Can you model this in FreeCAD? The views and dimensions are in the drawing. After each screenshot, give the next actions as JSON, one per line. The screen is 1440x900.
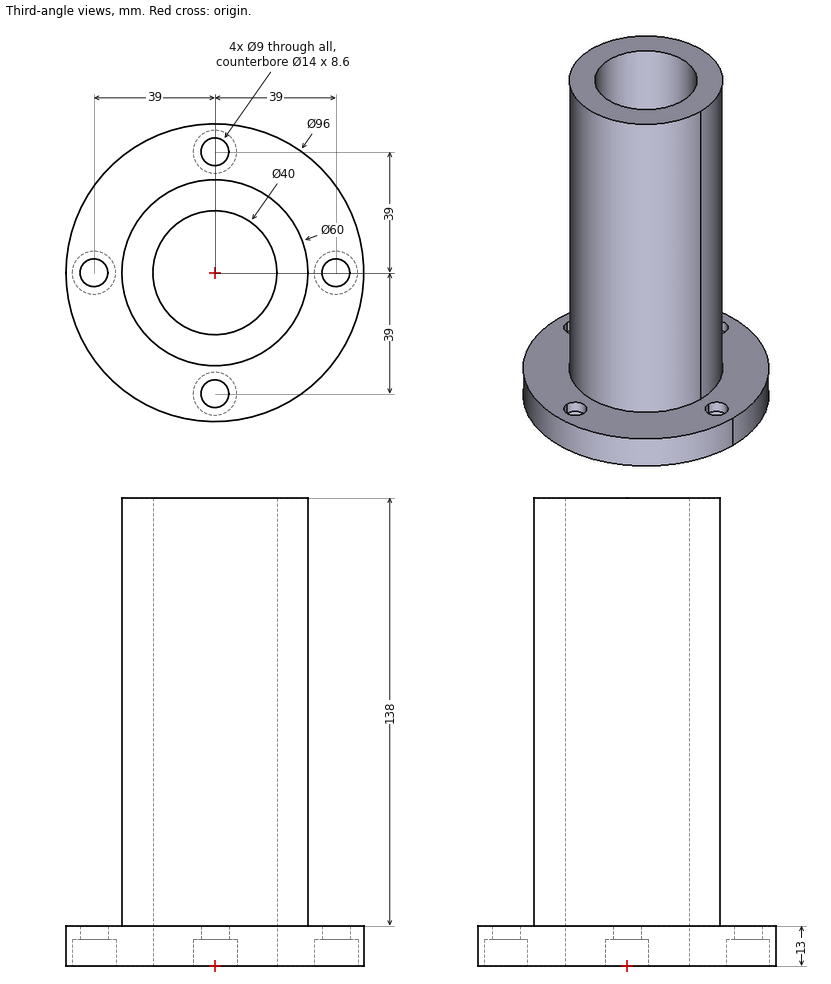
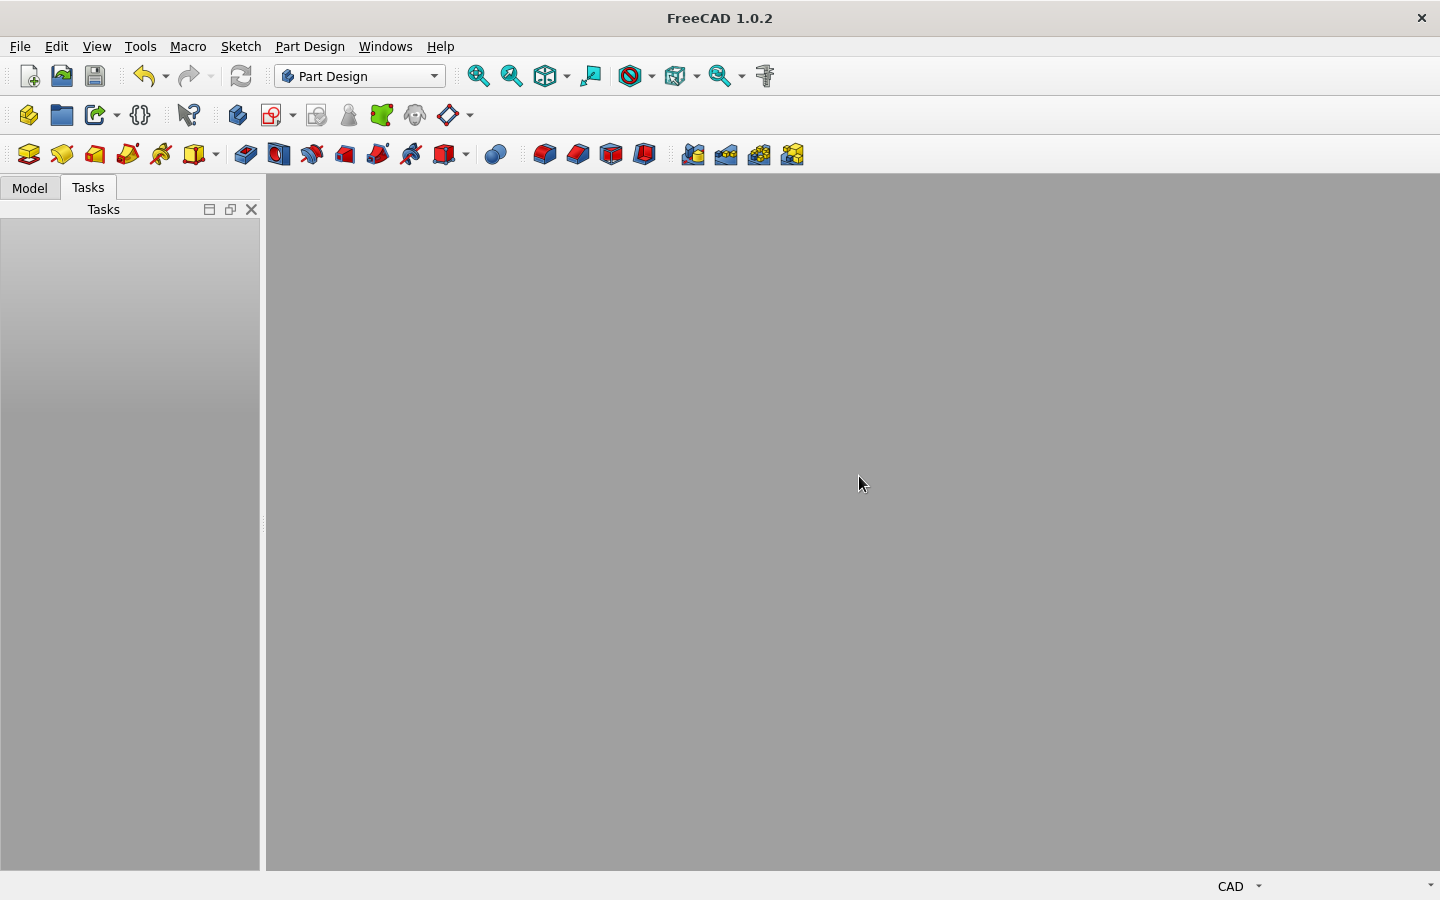
{"action": "key", "text": "ctrl+n"}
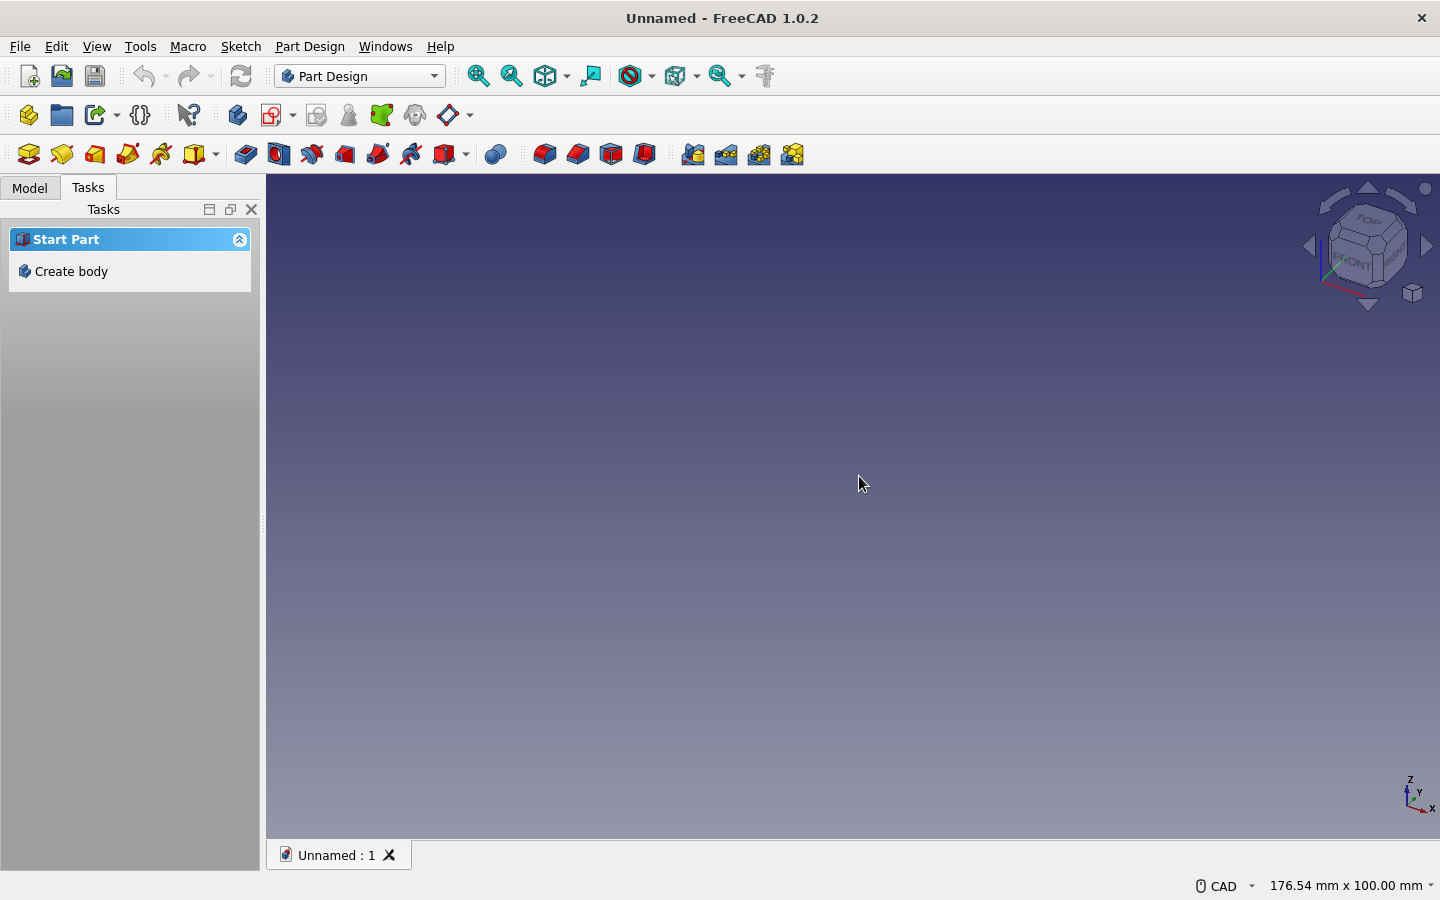
{"action": "left_click", "coordinate": [270, 116]}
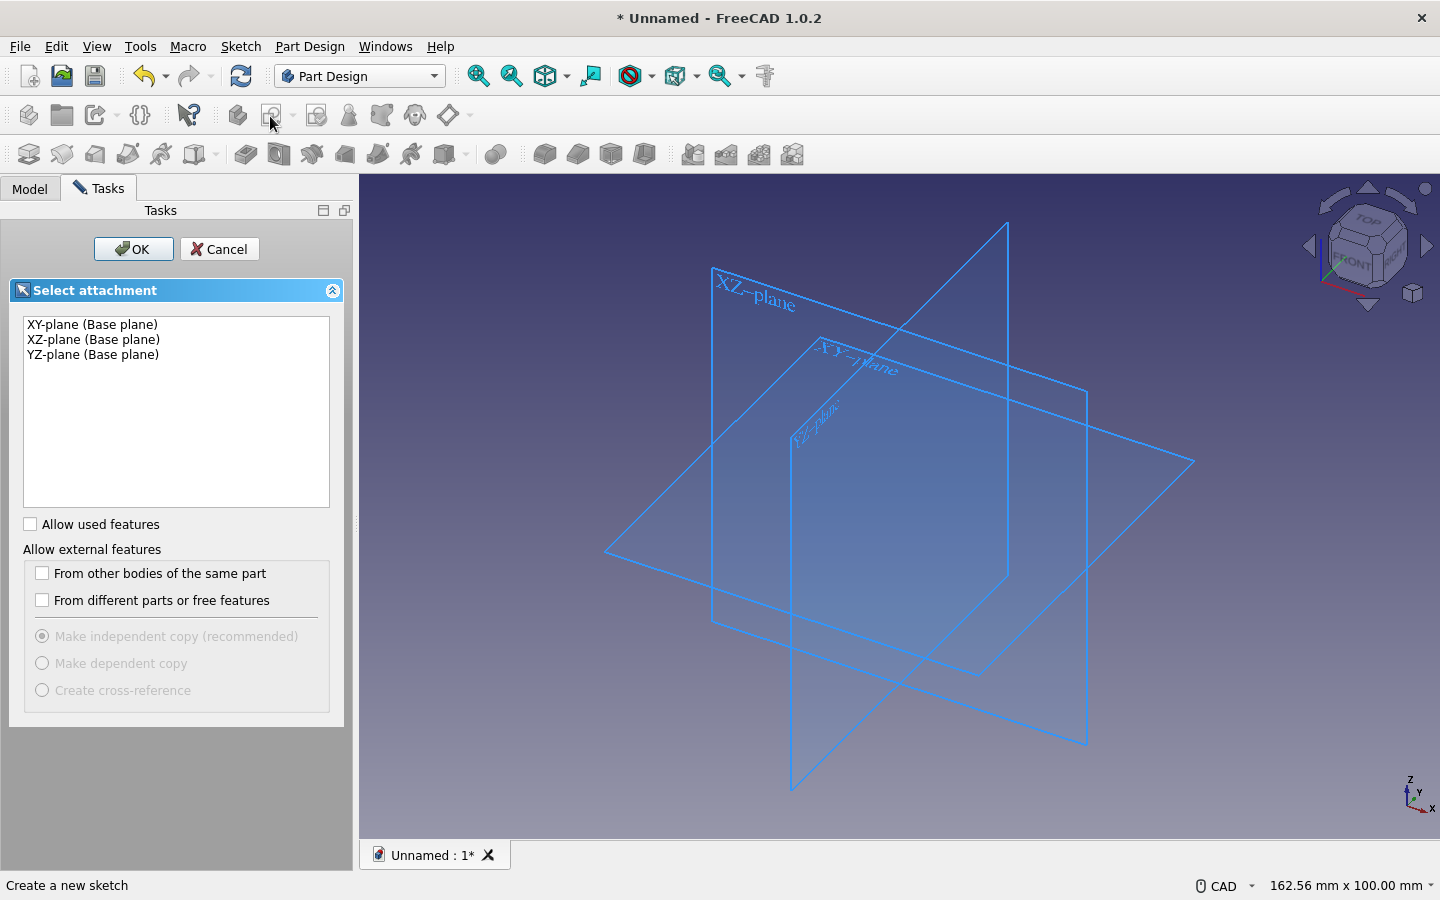
{"action": "left_click", "coordinate": [84, 324]}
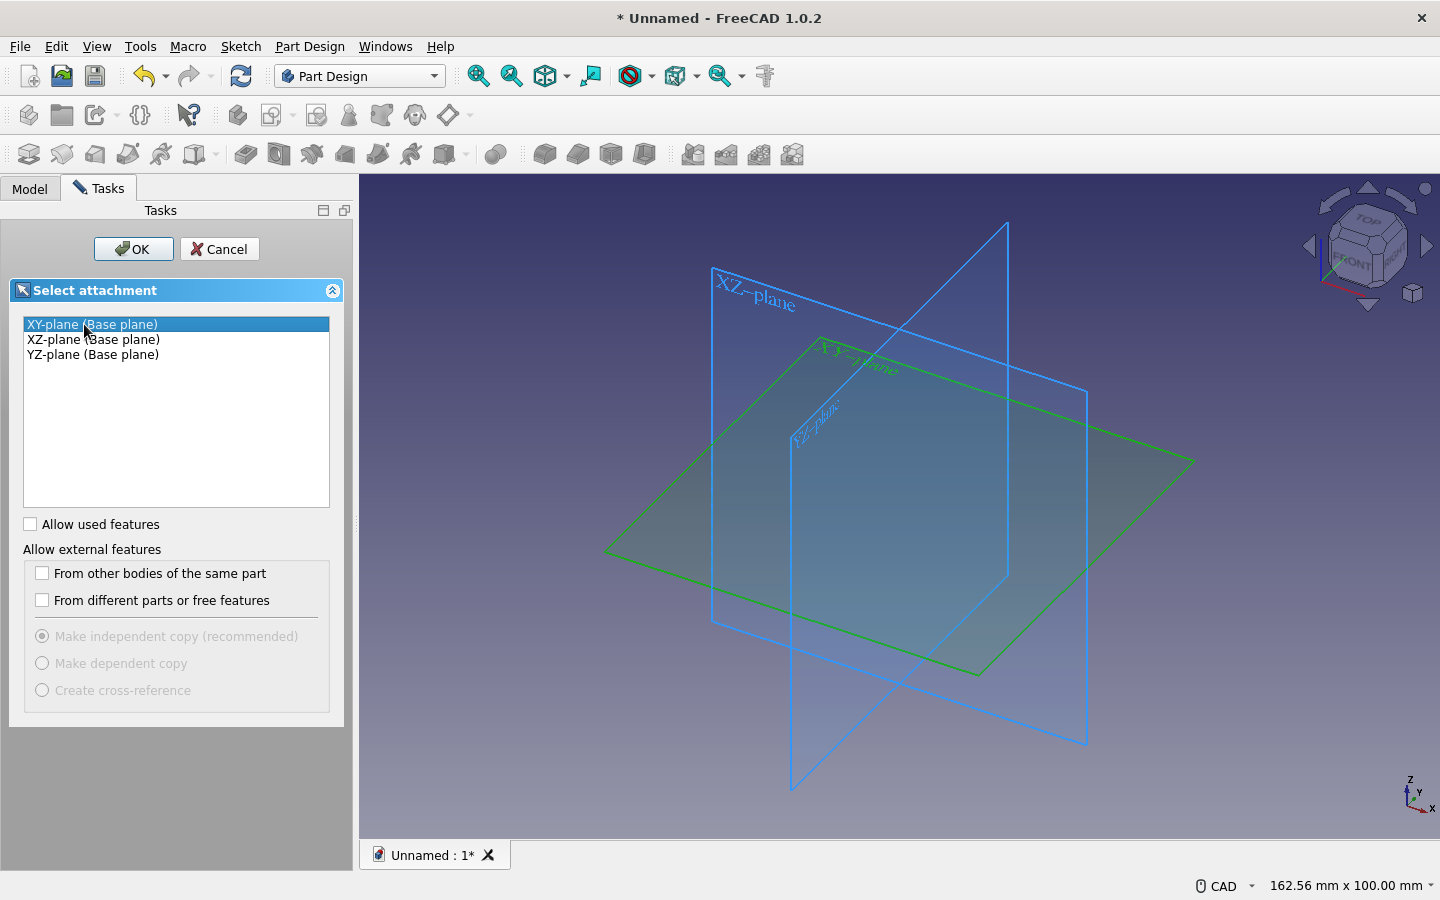
{"action": "left_click", "coordinate": [134, 249]}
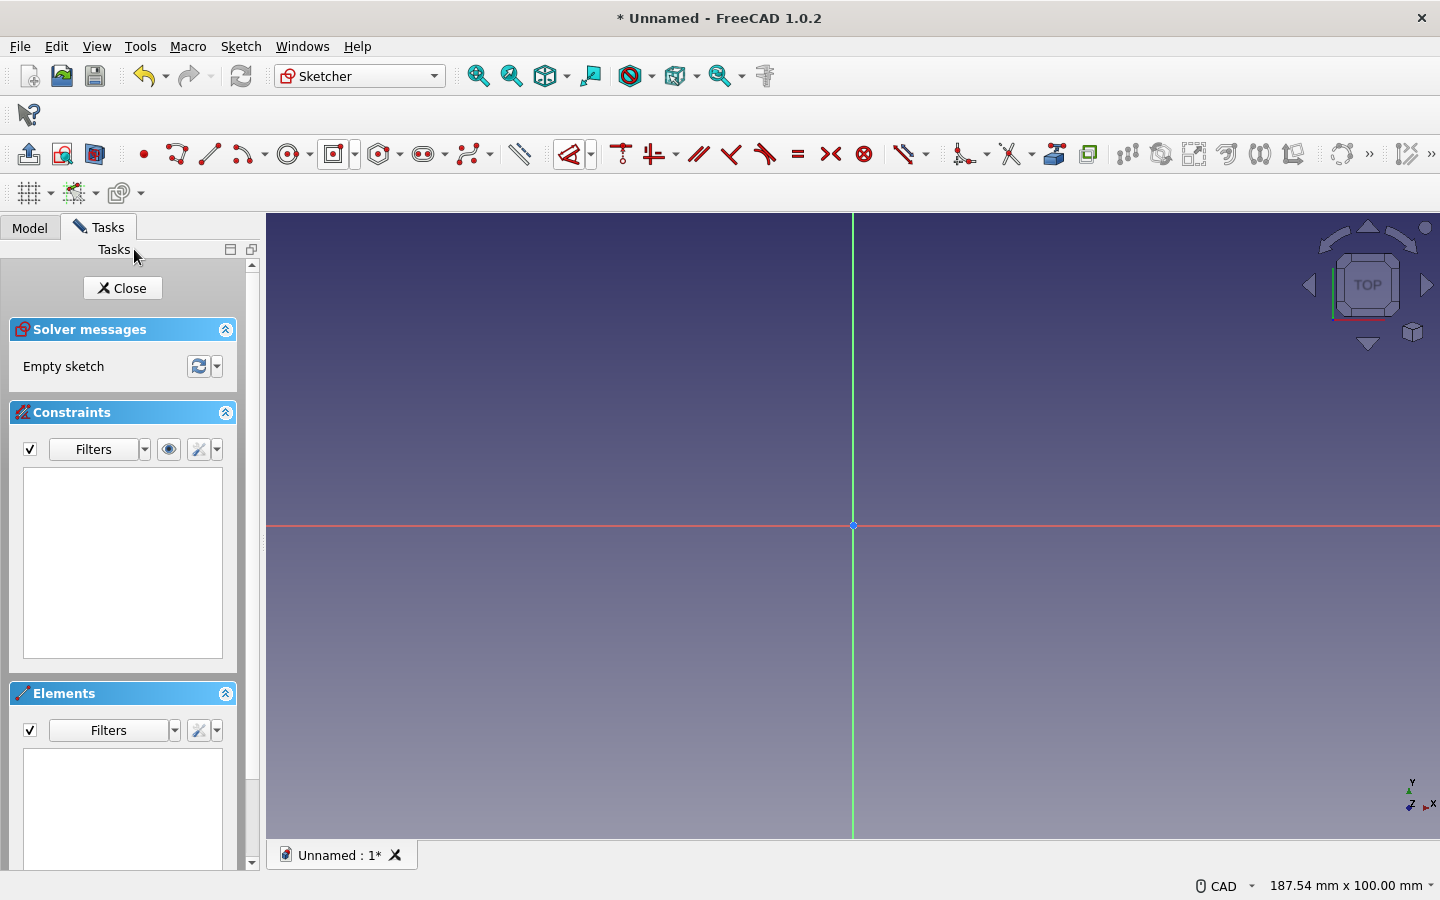
{"action": "scroll", "coordinate": [645, 526], "scroll_direction": "down", "scroll_amount": 2}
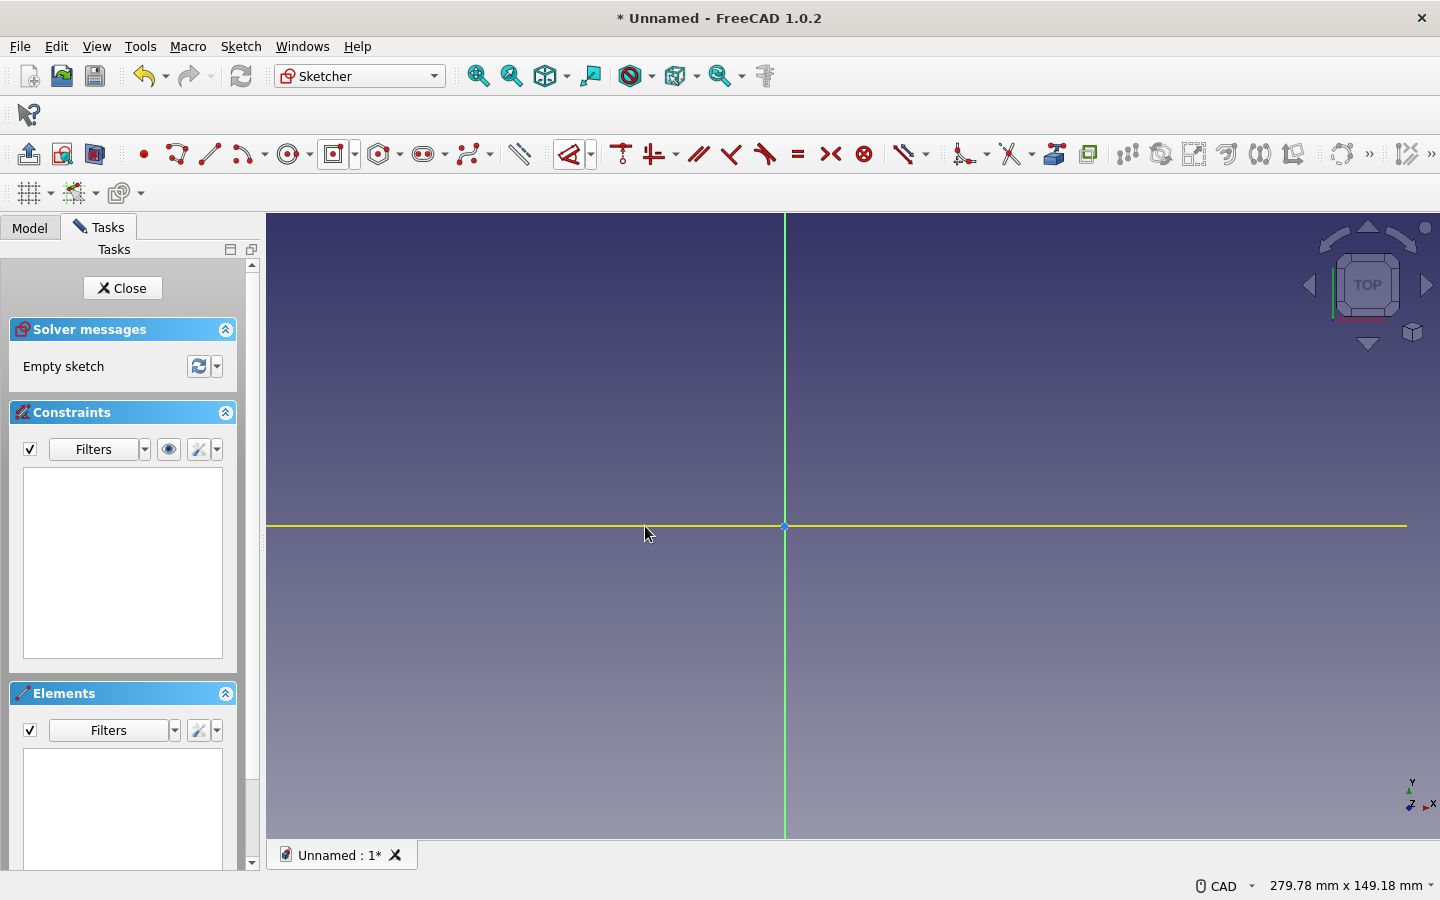
{"action": "left_click", "coordinate": [288, 154]}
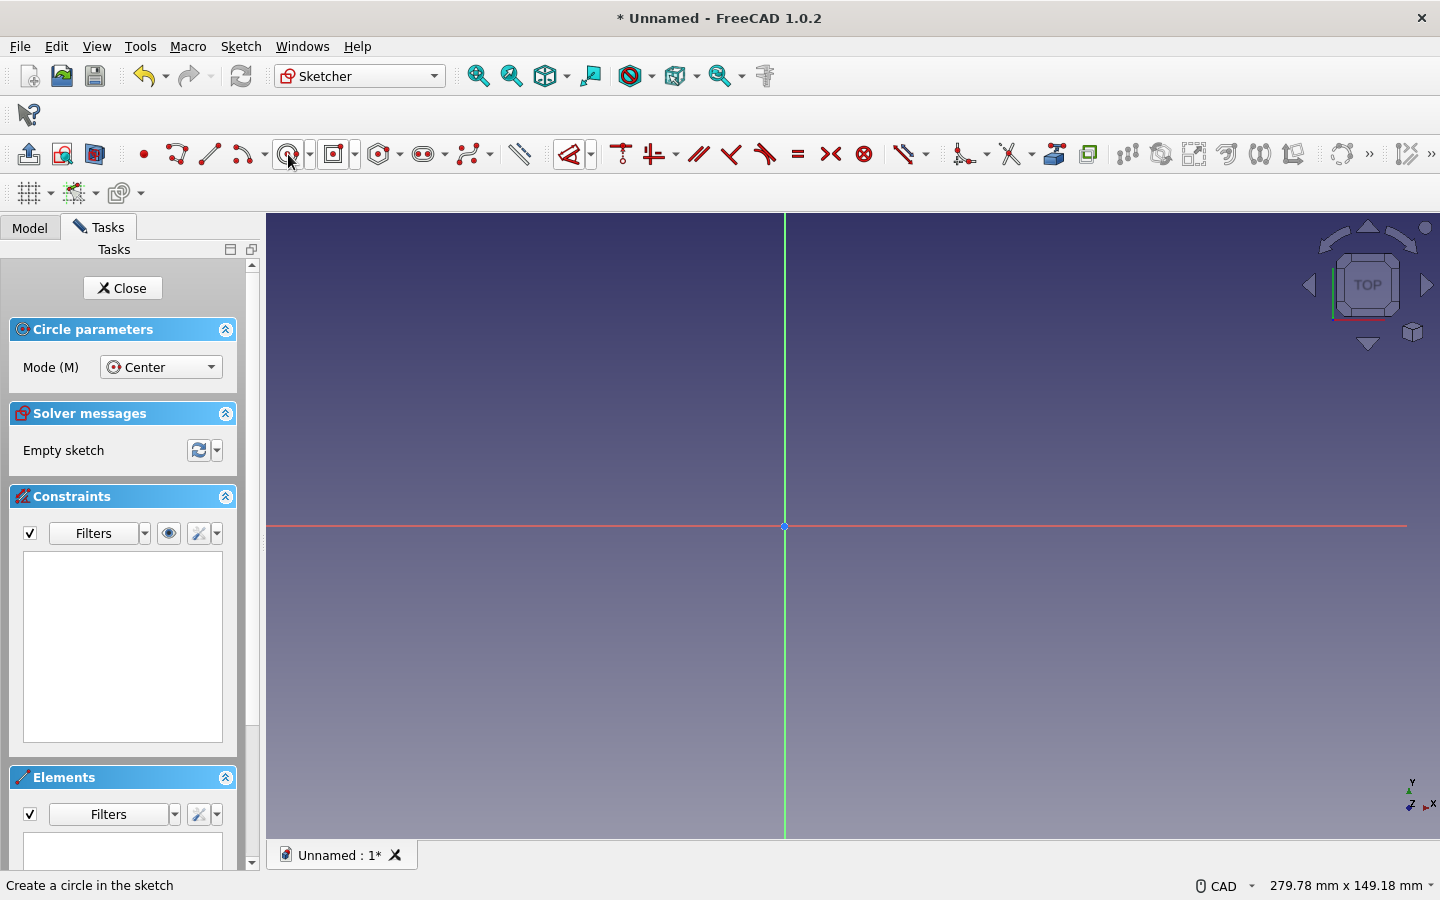
{"action": "left_click", "coordinate": [785, 526]}
{"action": "mouse_move", "coordinate": [927, 384]}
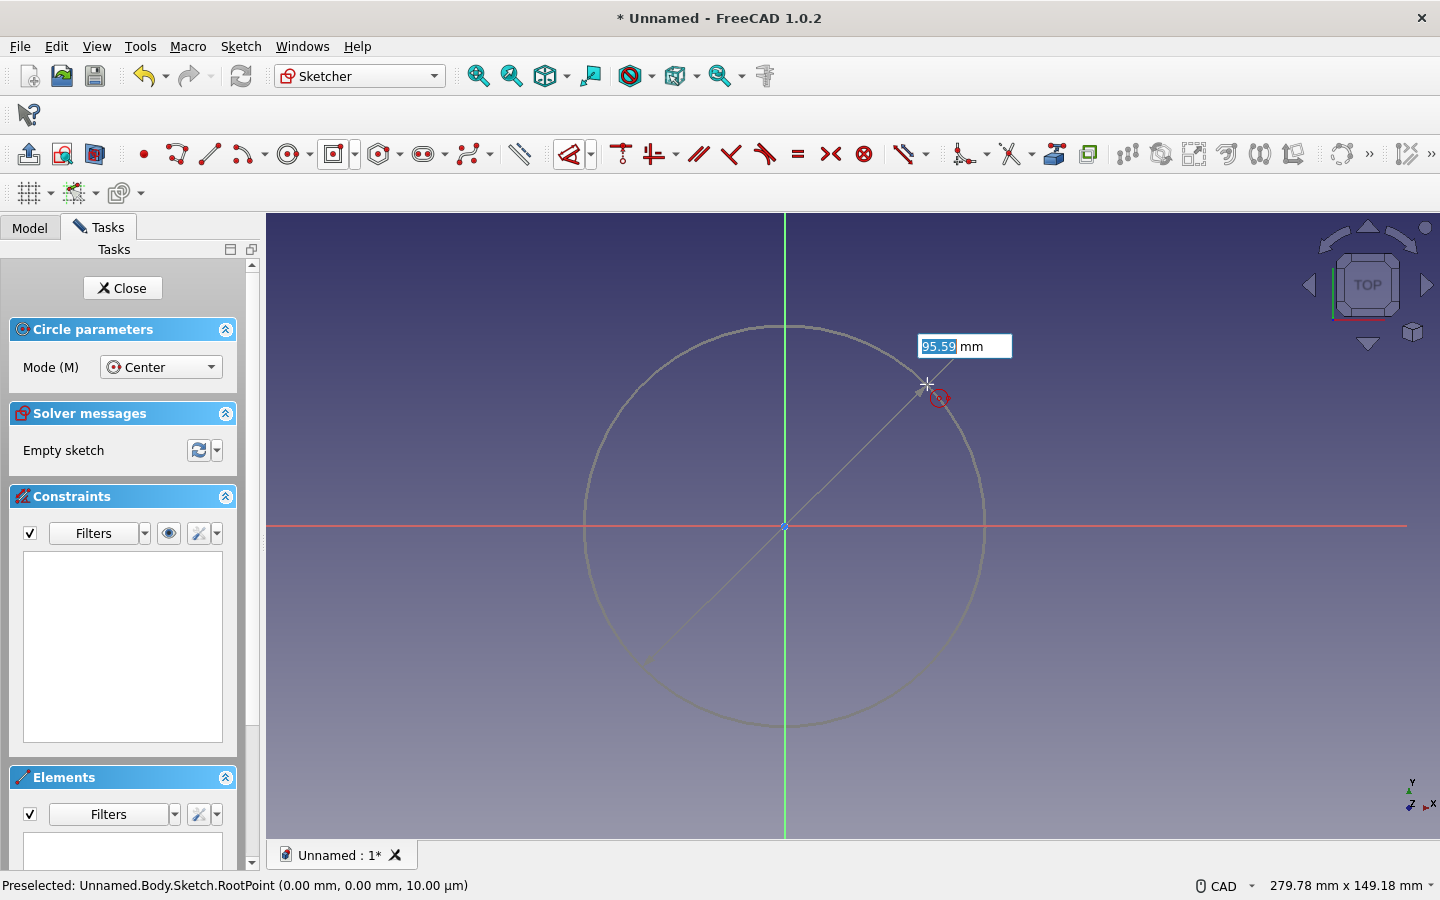
{"action": "type", "text": "96"}
{"action": "key", "text": "Return"}
{"action": "key", "text": "Escape"}